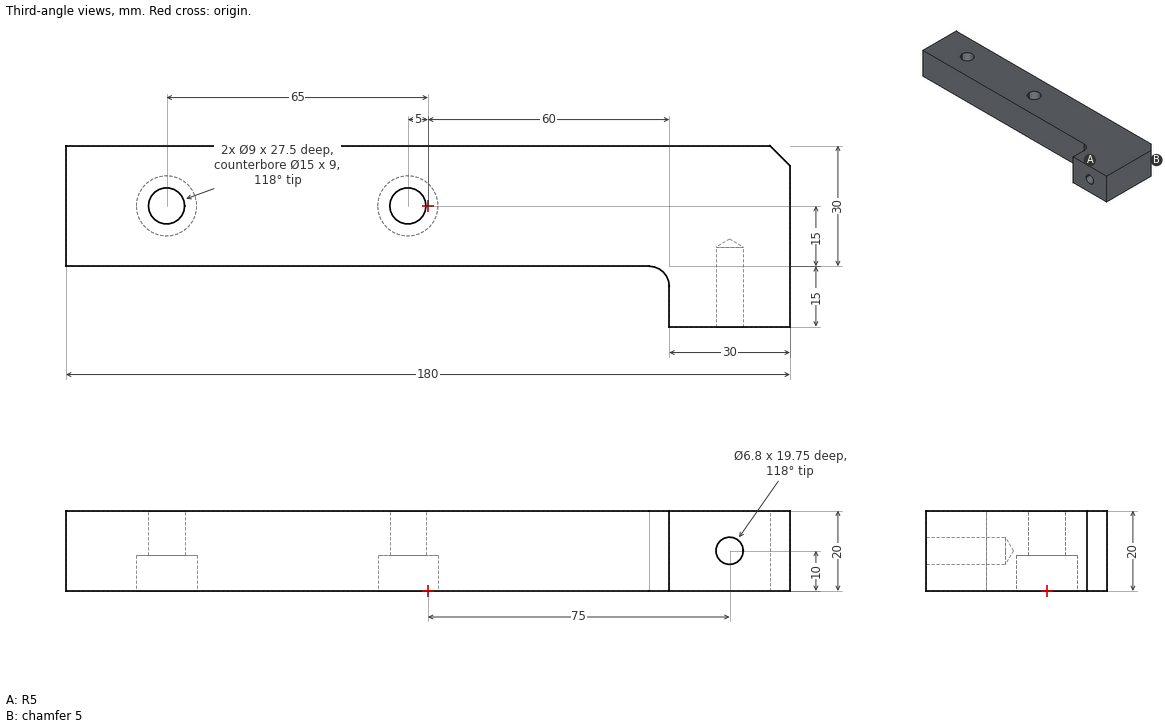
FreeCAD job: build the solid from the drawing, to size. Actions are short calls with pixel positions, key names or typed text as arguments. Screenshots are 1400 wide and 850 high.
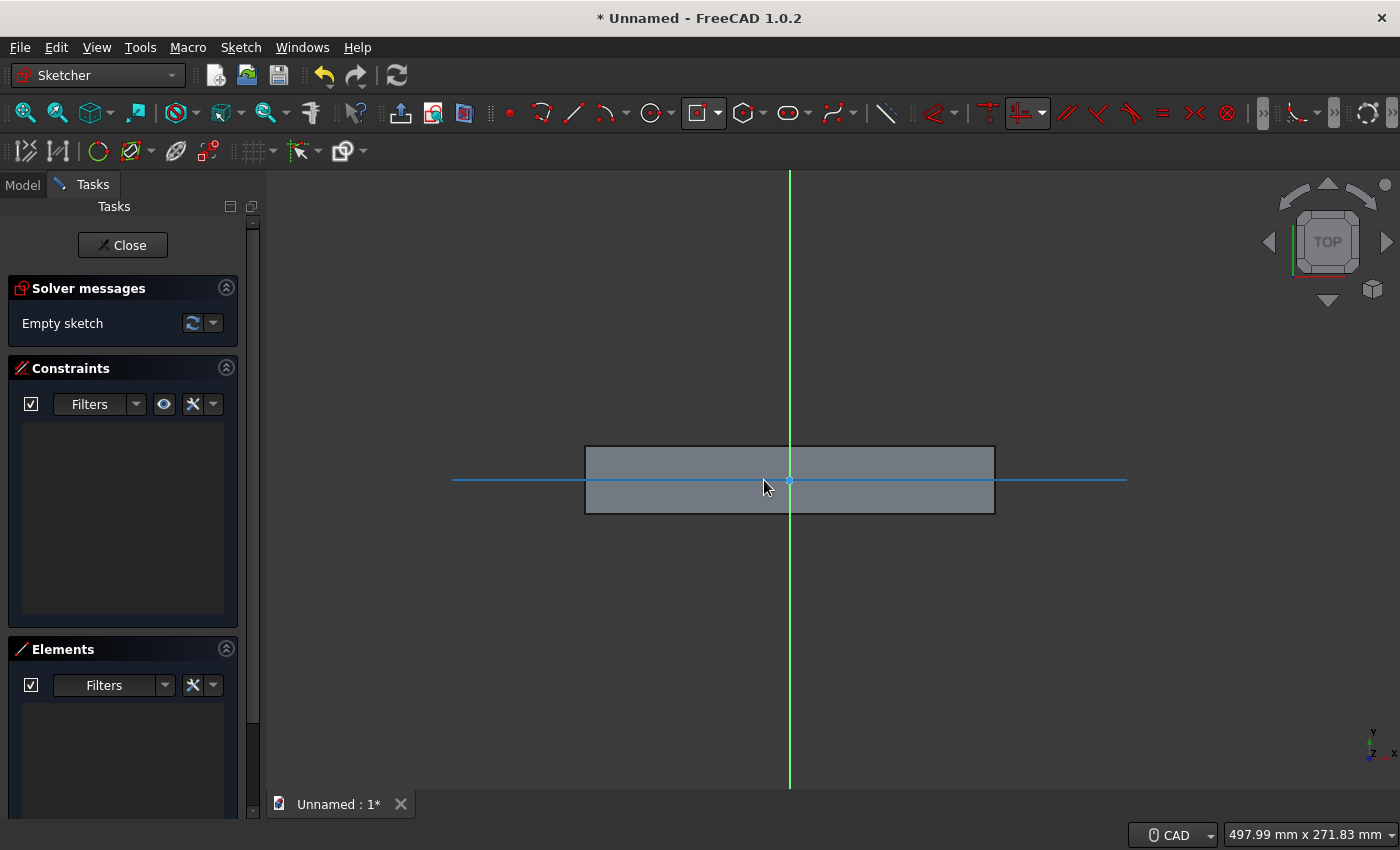
scroll(985, 538, up, 11)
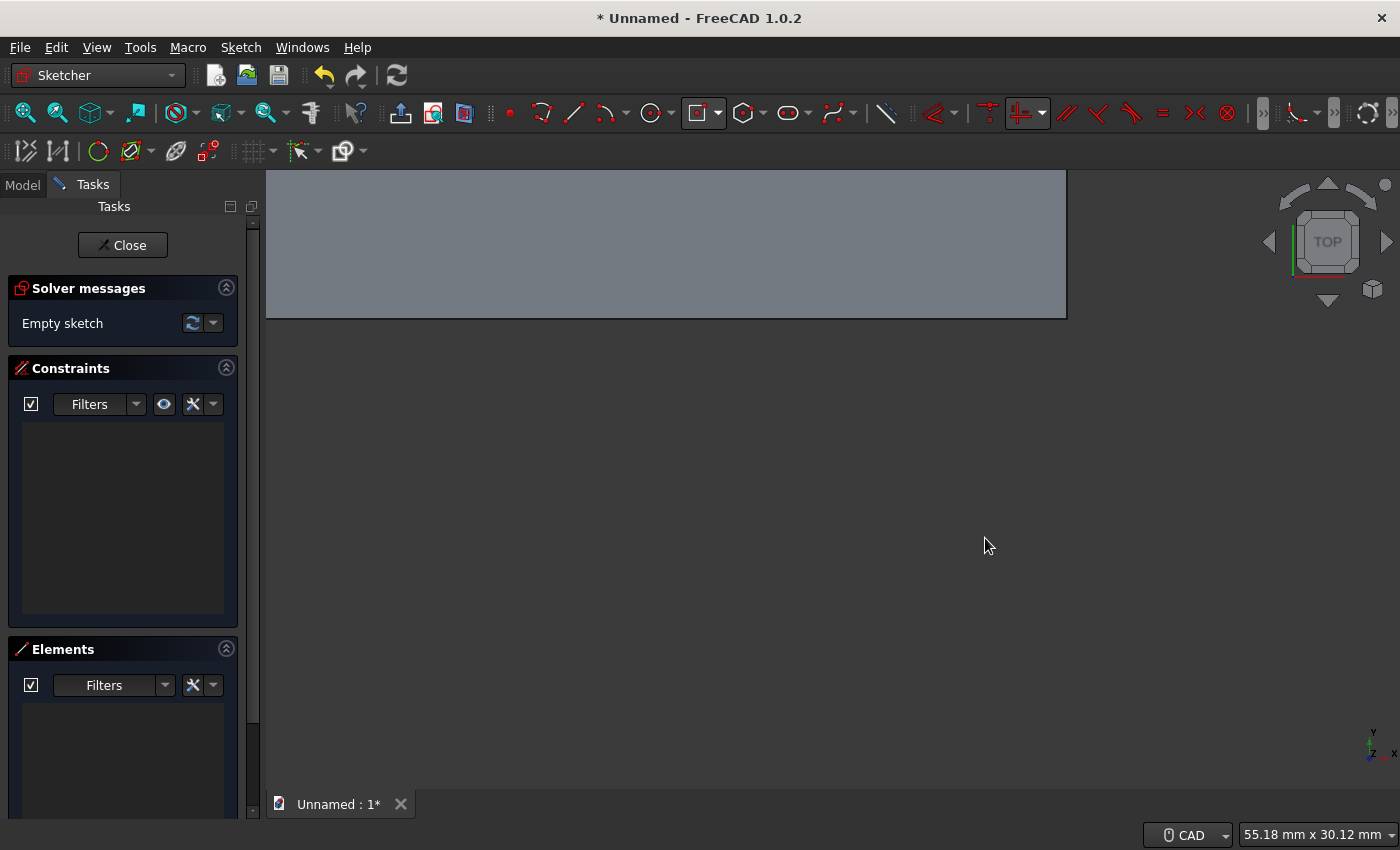
key(g)
key(r)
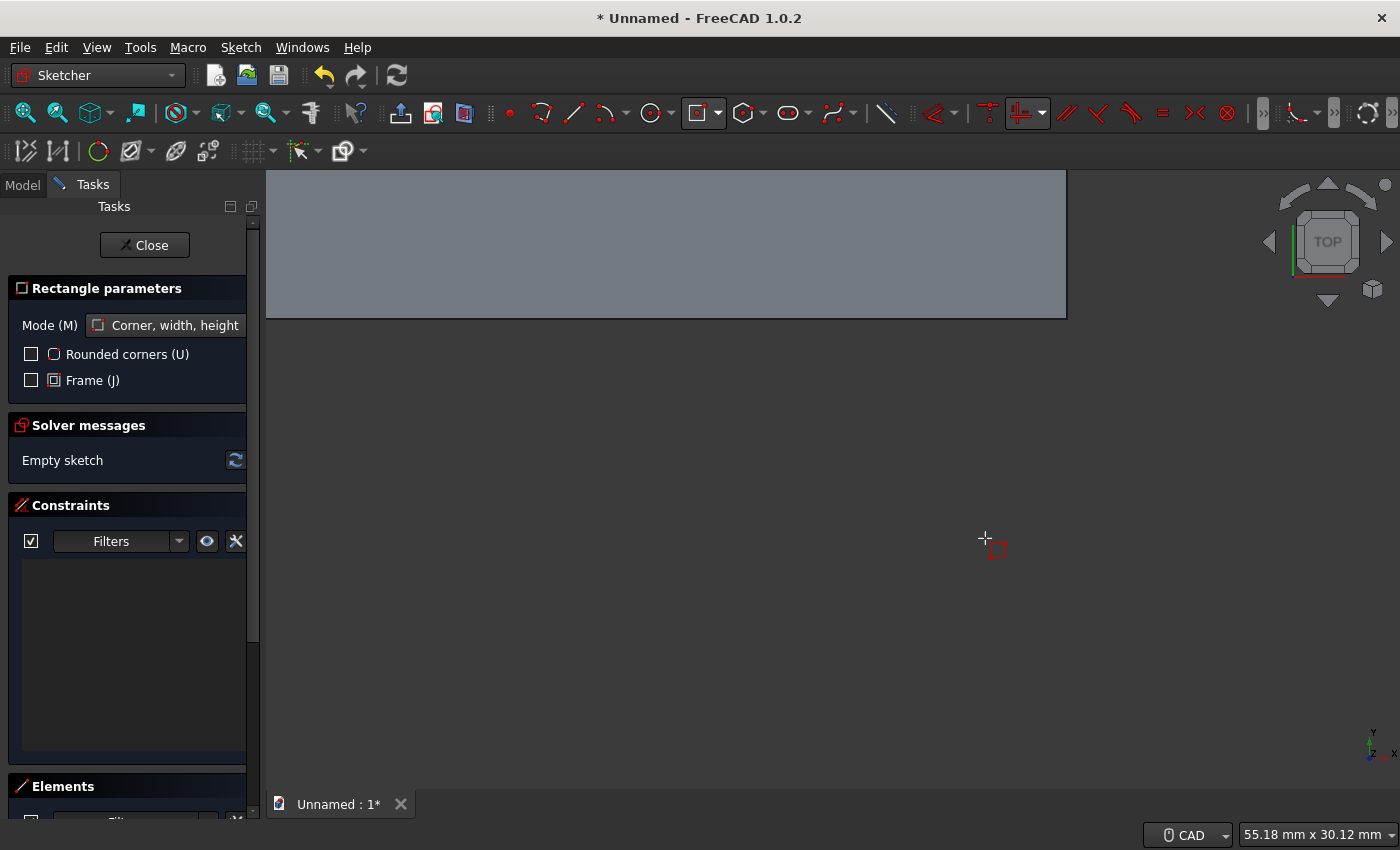
click(450, 319)
move(1067, 628)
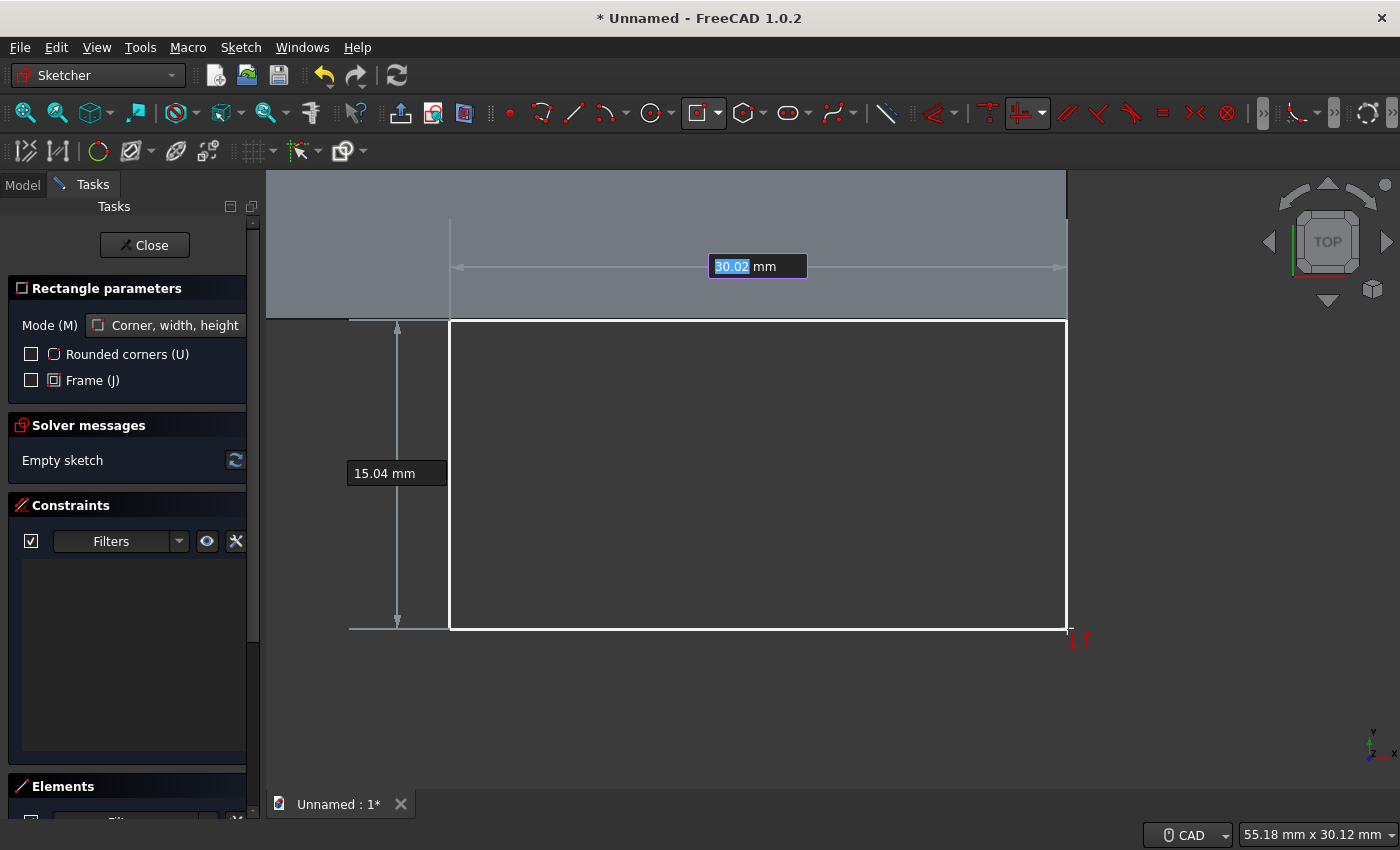
text(30)
key(Tab)
text(15)
key(Return)
key(Escape)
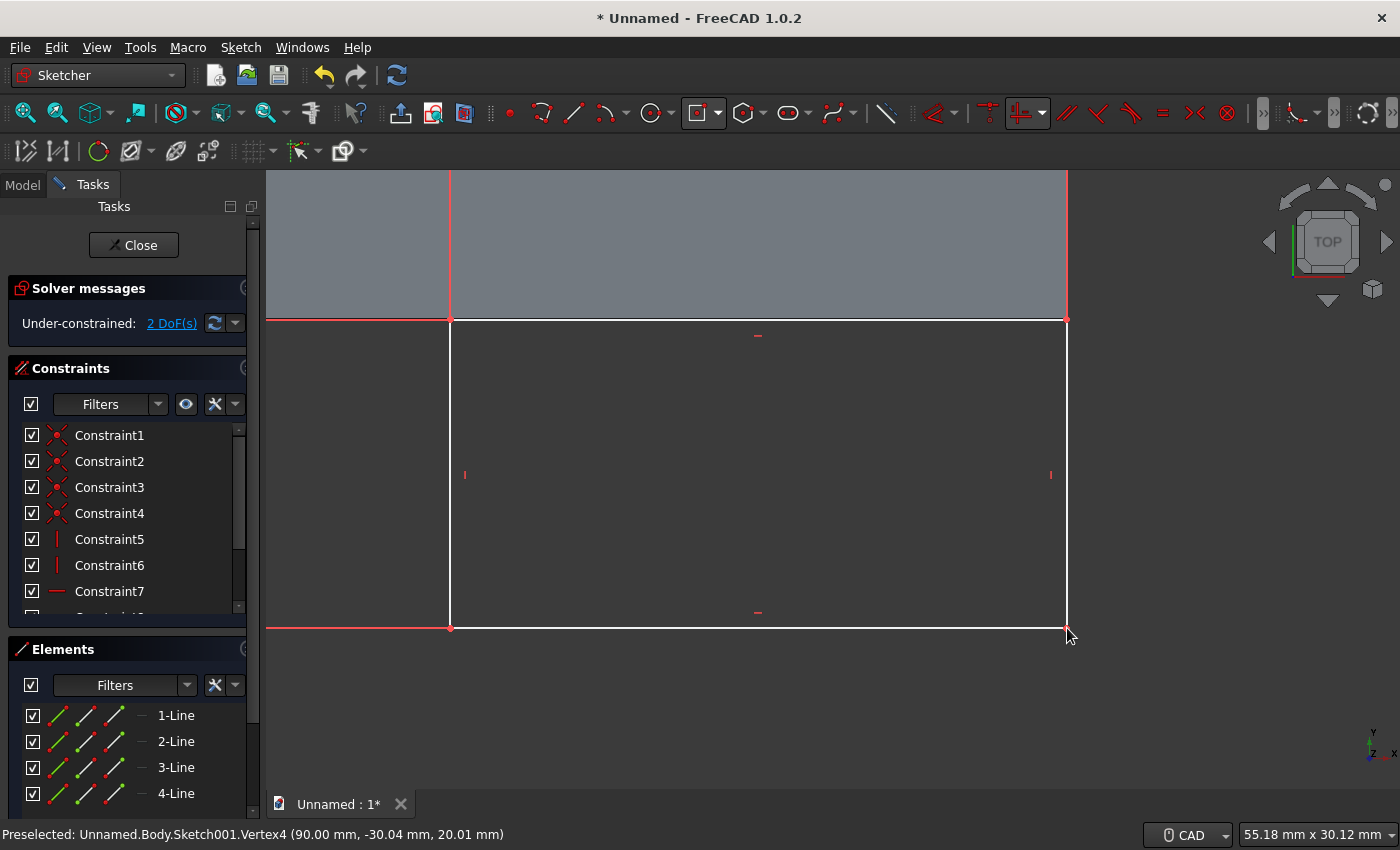
key(d)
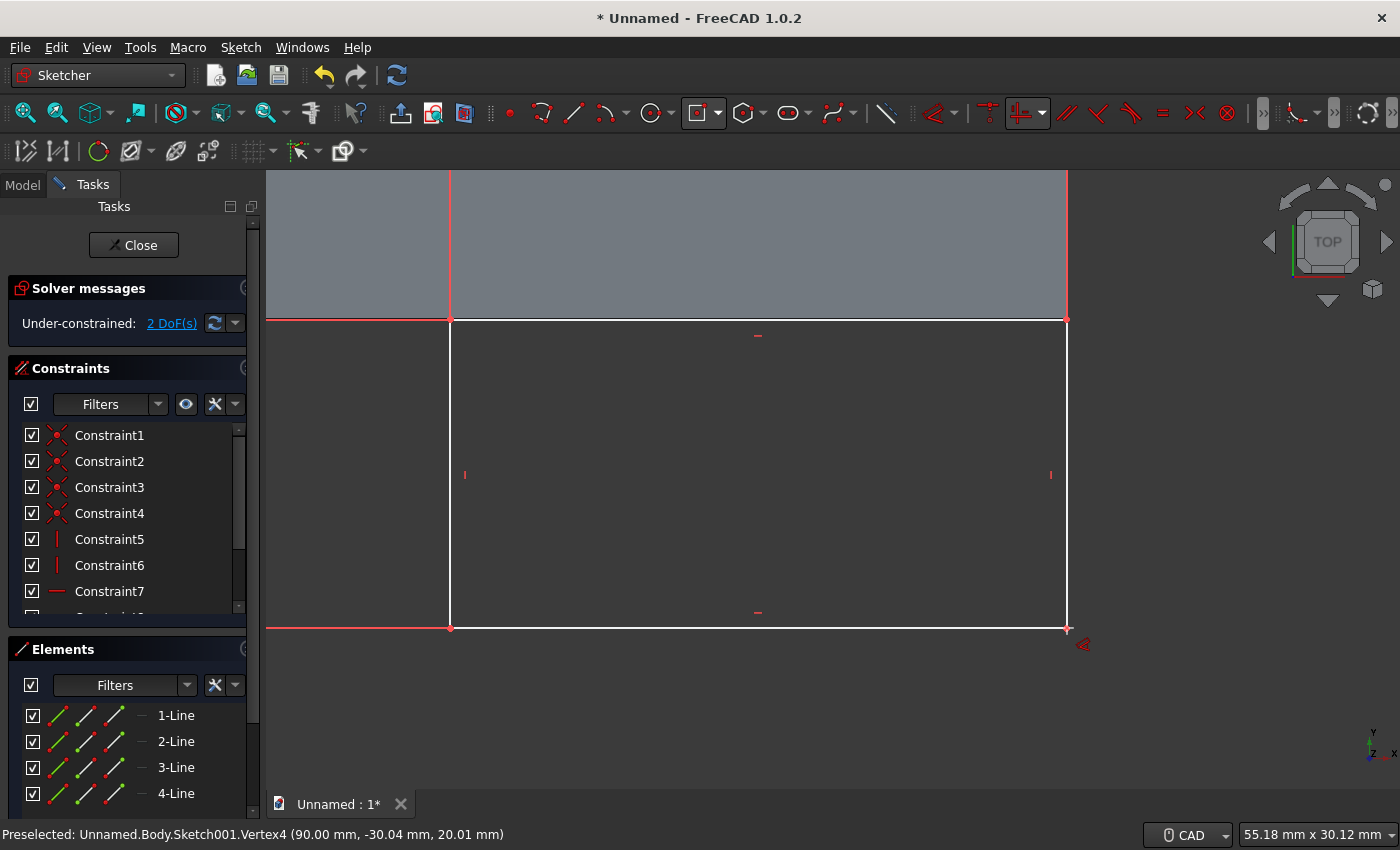
click(450, 320)
click(372, 354)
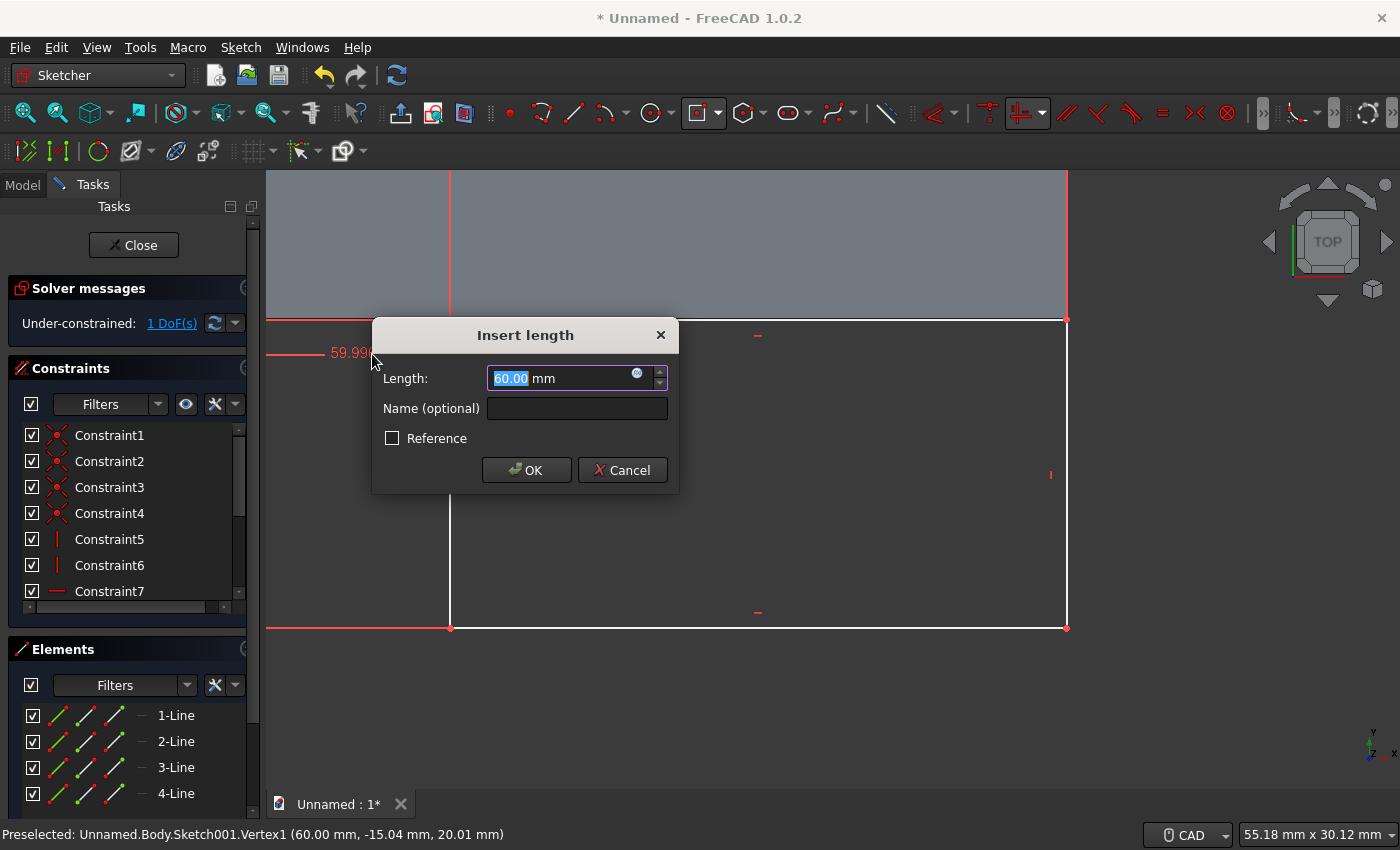
text(60)
key(Return)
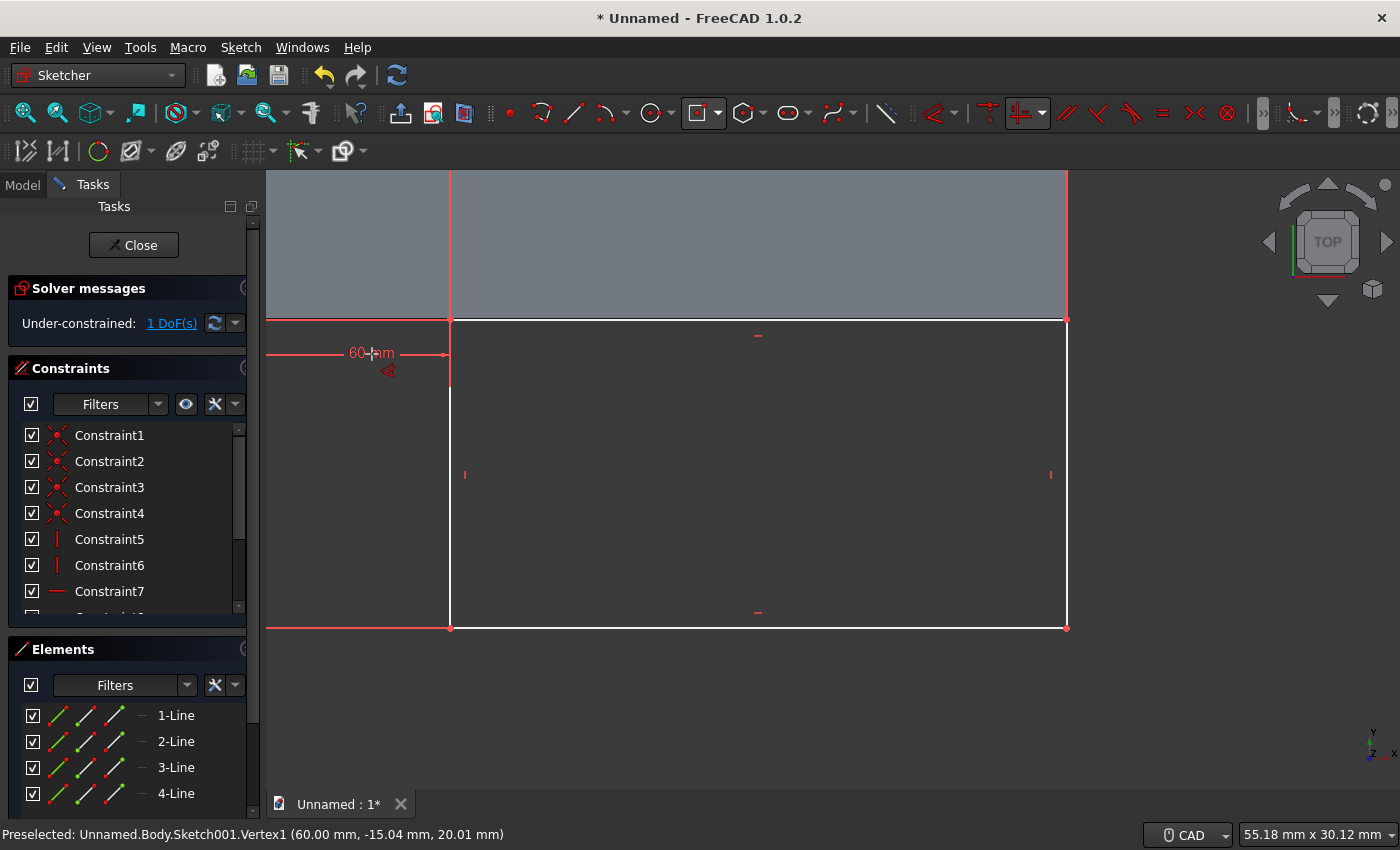
click(450, 320)
click(484, 259)